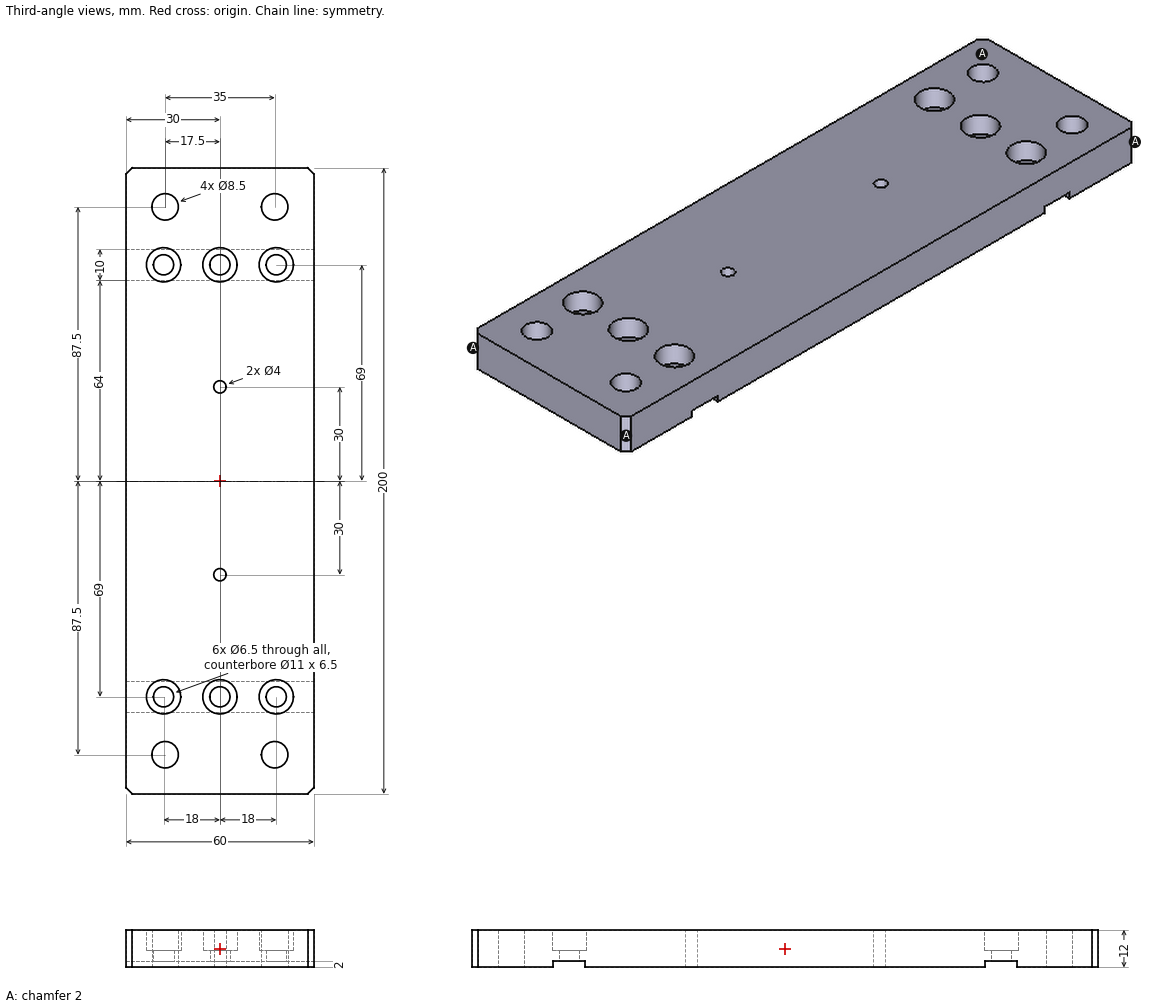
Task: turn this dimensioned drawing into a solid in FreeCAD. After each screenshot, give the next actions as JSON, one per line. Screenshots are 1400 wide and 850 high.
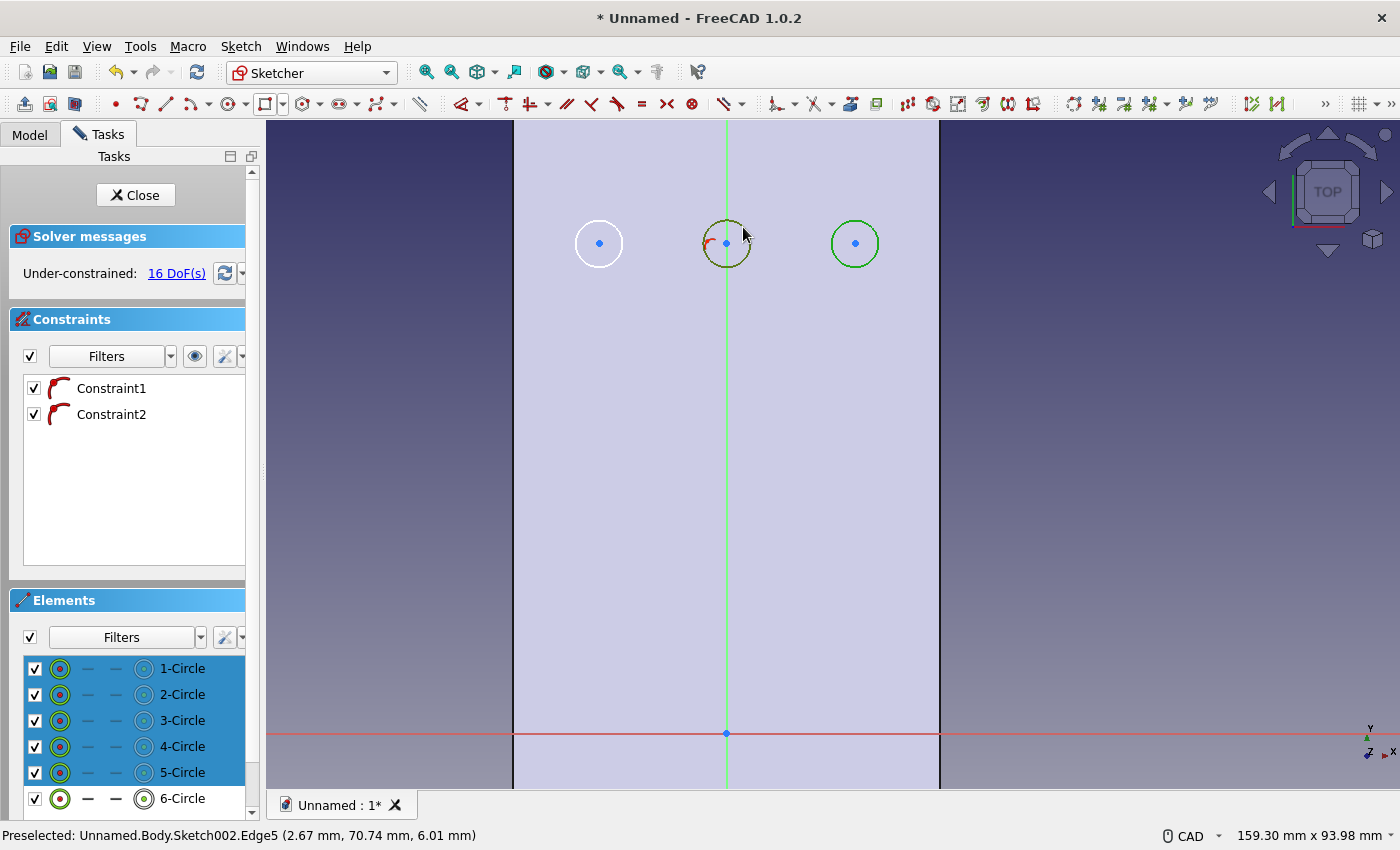
{"action": "left_click", "coordinate": [616, 227]}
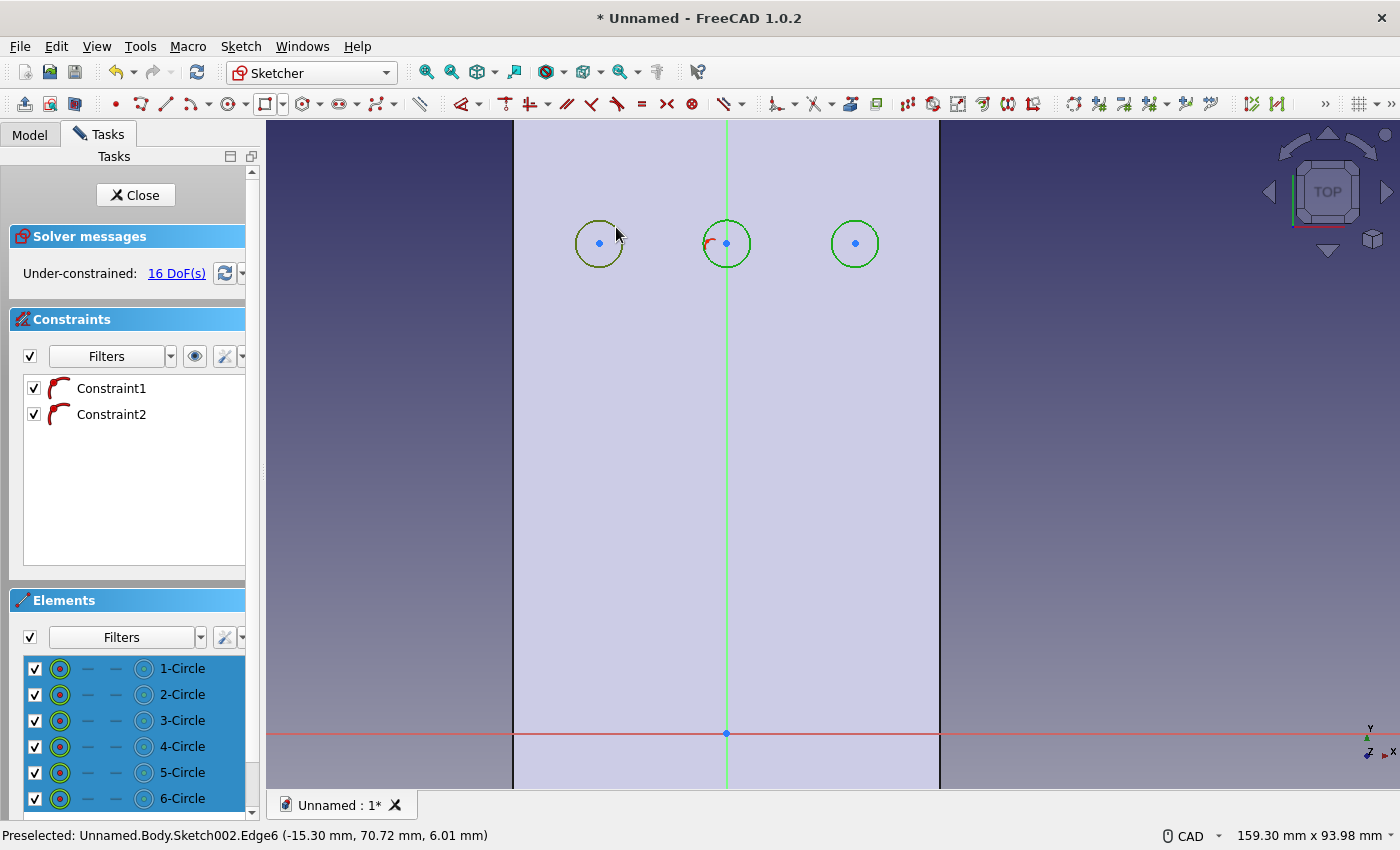
{"action": "left_click", "coordinate": [642, 104]}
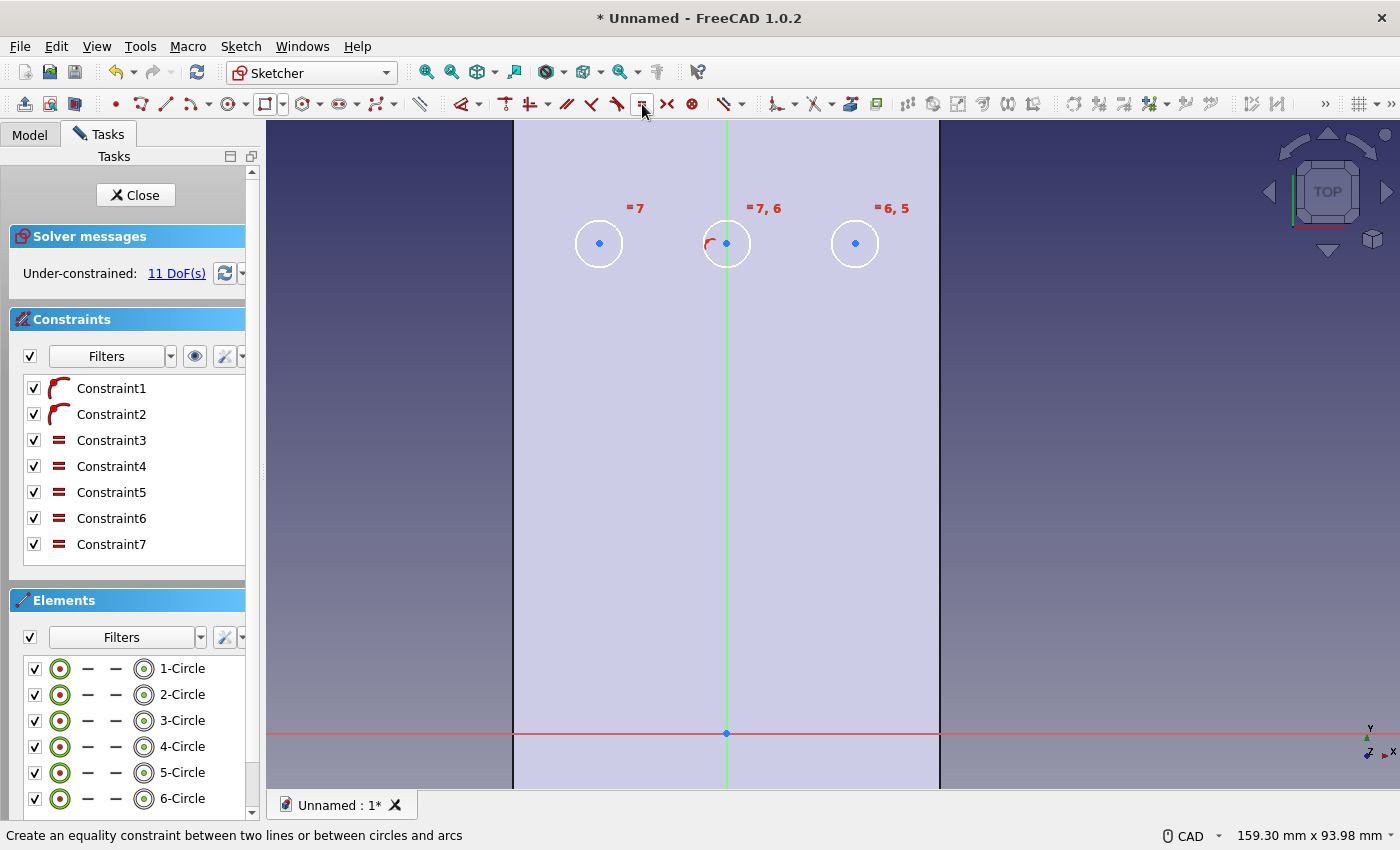
{"action": "scroll", "coordinate": [795, 227], "scroll_direction": "down", "scroll_amount": 4}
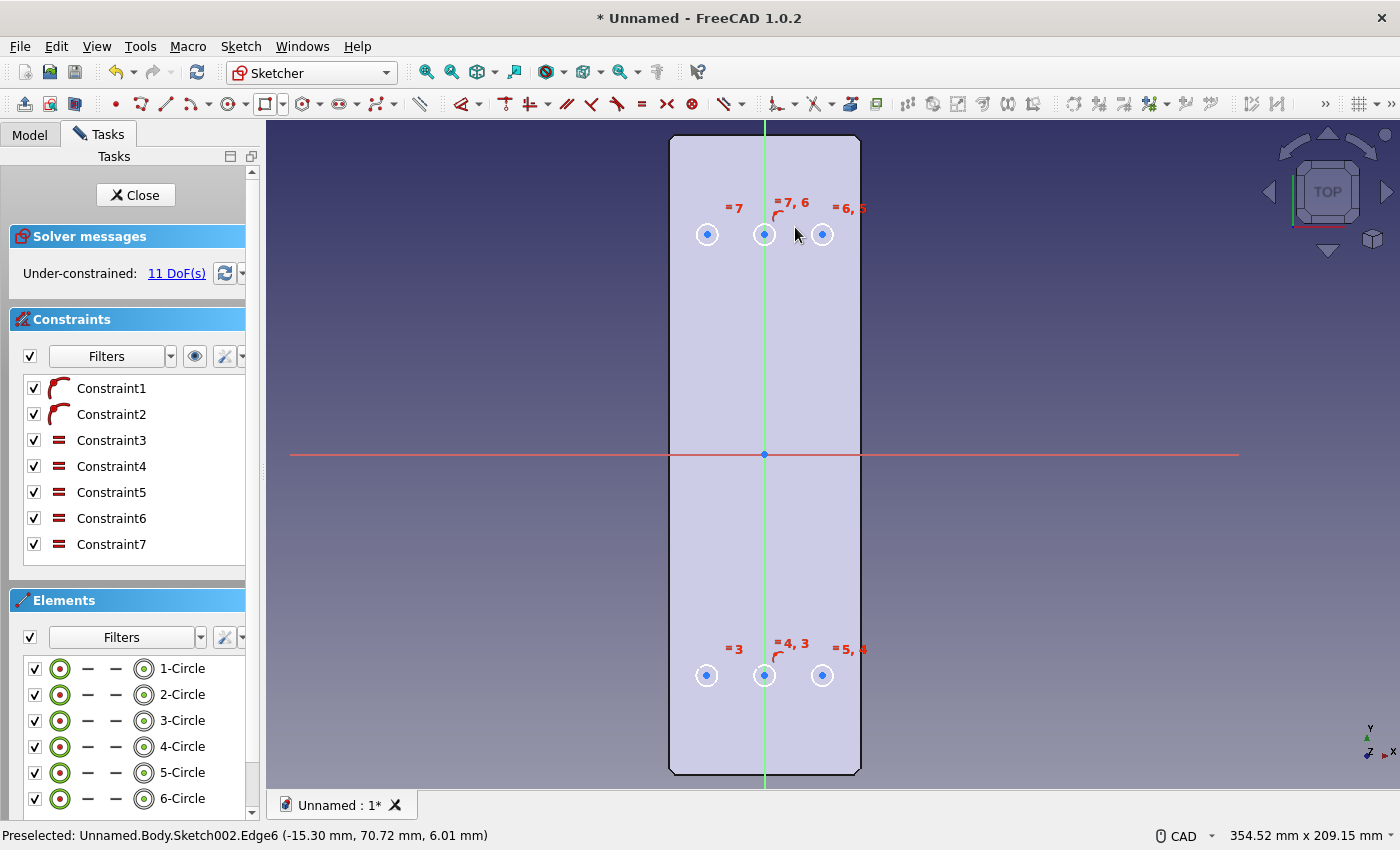
{"action": "left_click", "coordinate": [707, 676]}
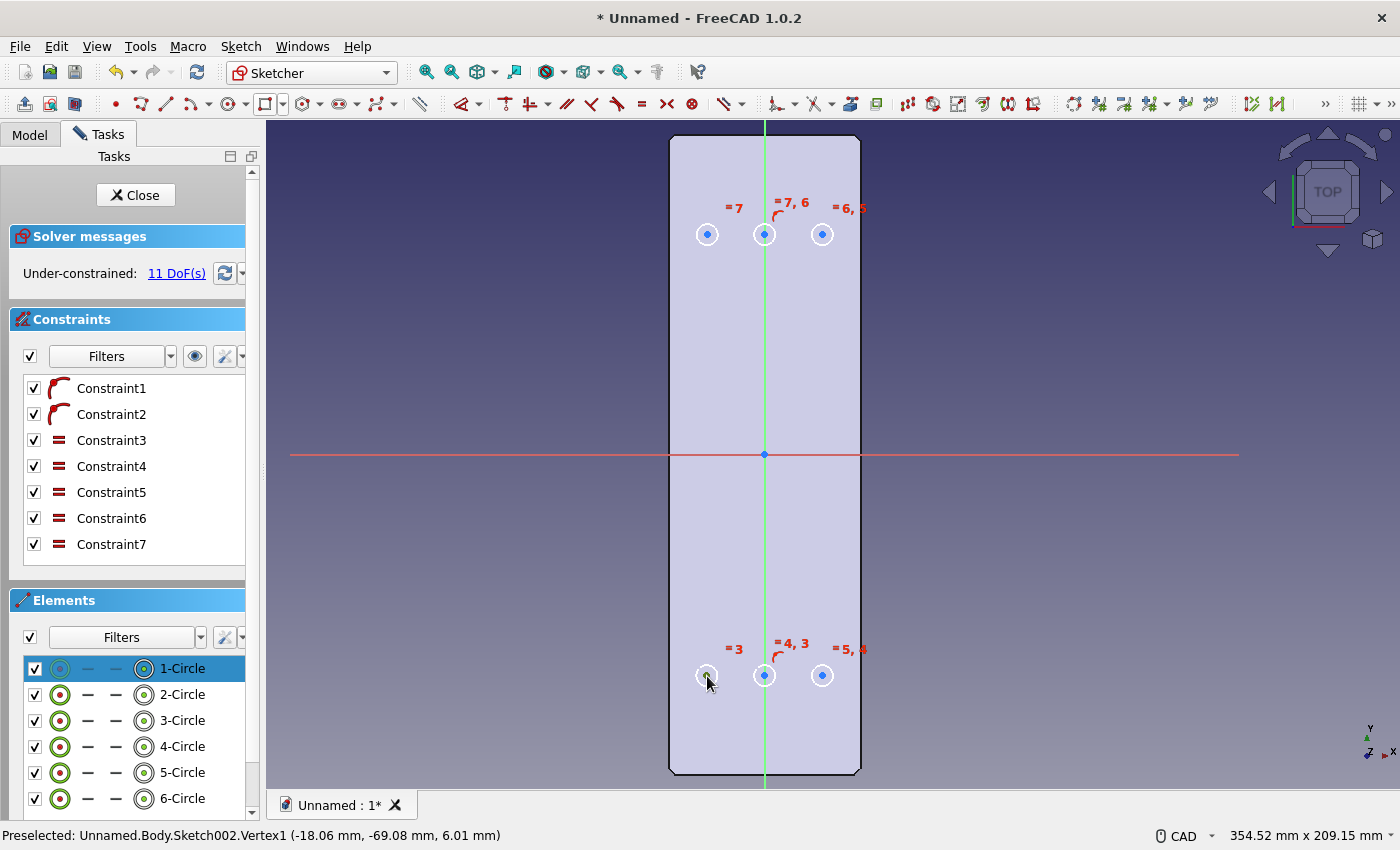
{"action": "left_click", "coordinate": [765, 676]}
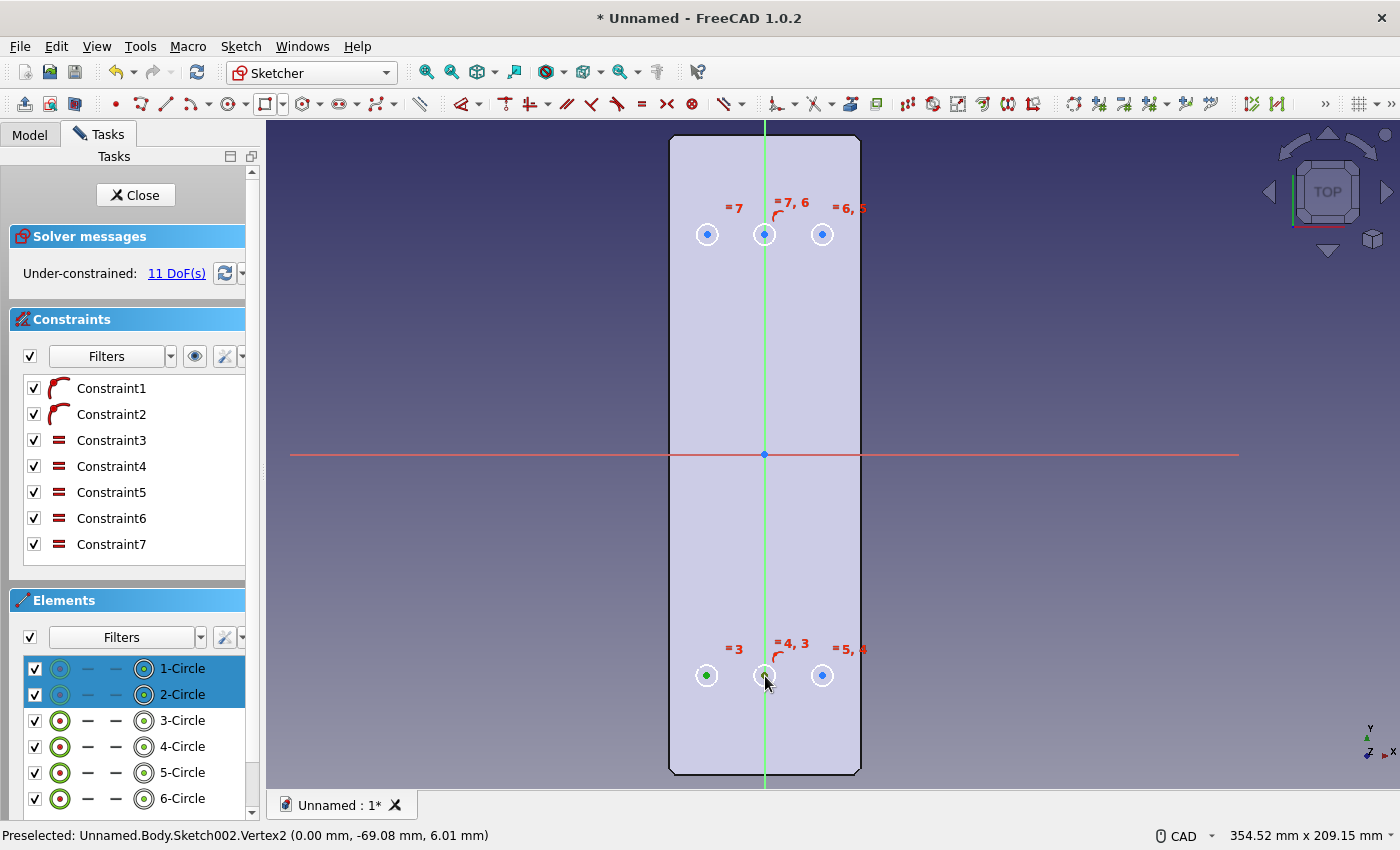
{"action": "left_click", "coordinate": [548, 104]}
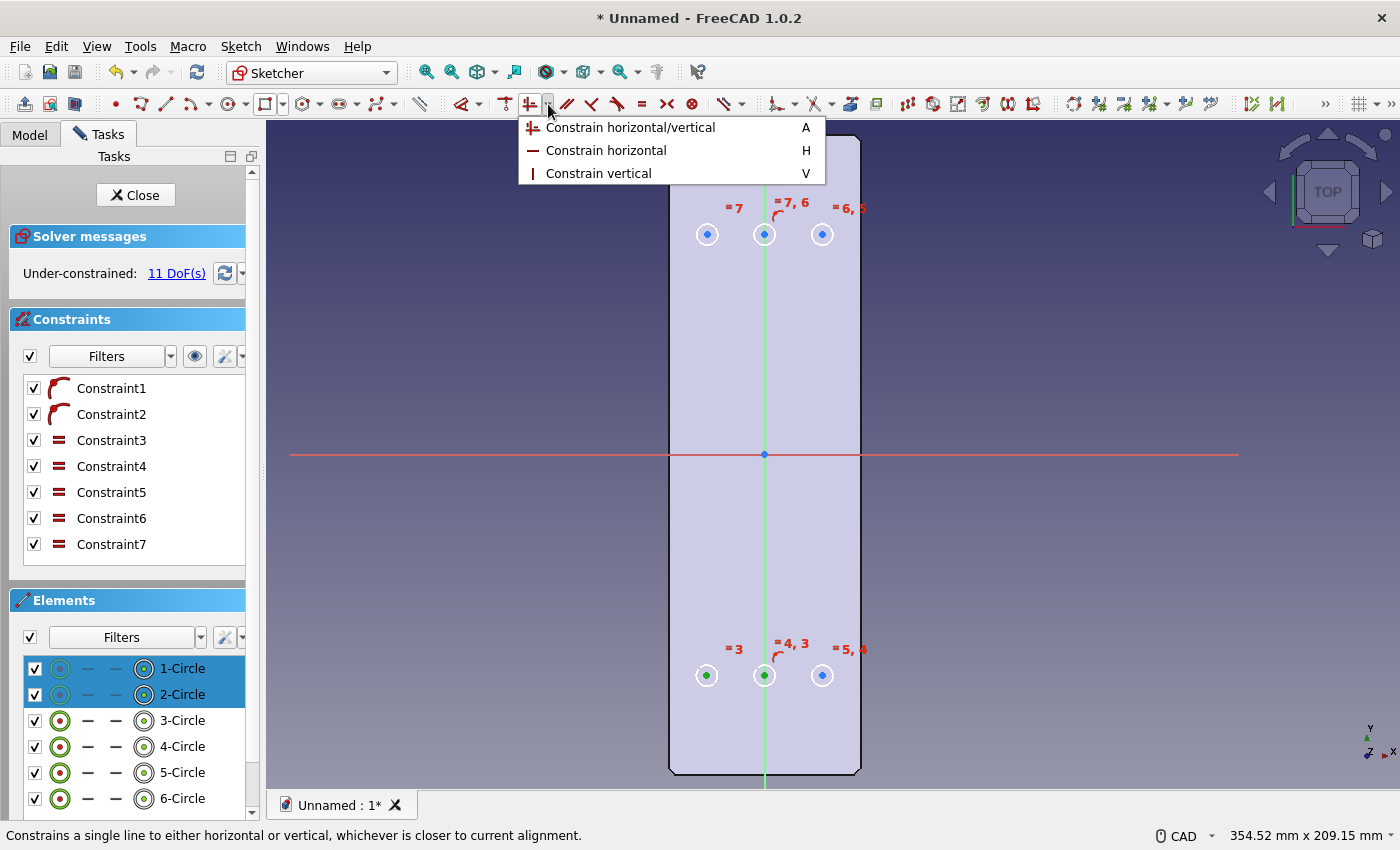
{"action": "left_click", "coordinate": [672, 150]}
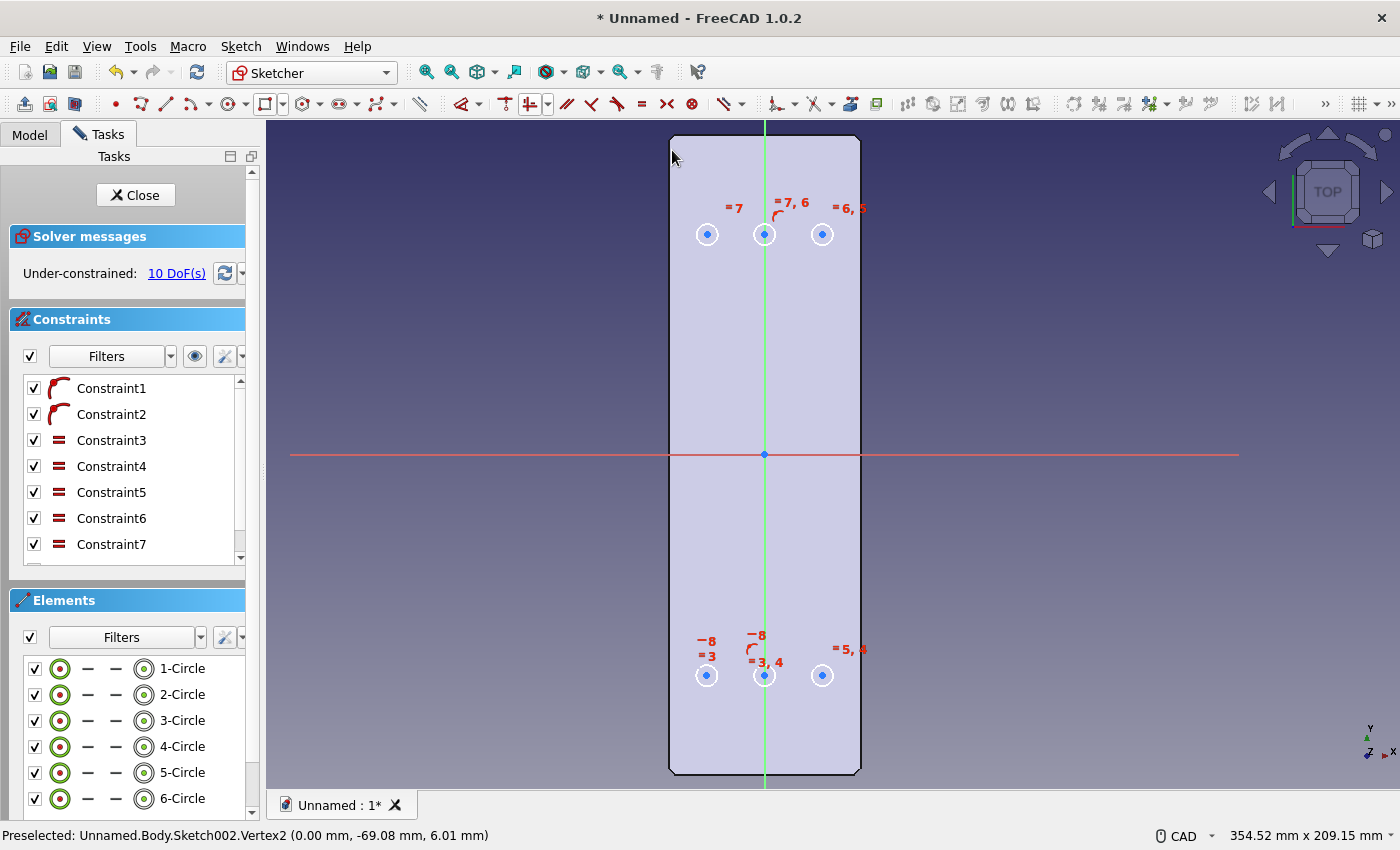
{"action": "left_click", "coordinate": [765, 676]}